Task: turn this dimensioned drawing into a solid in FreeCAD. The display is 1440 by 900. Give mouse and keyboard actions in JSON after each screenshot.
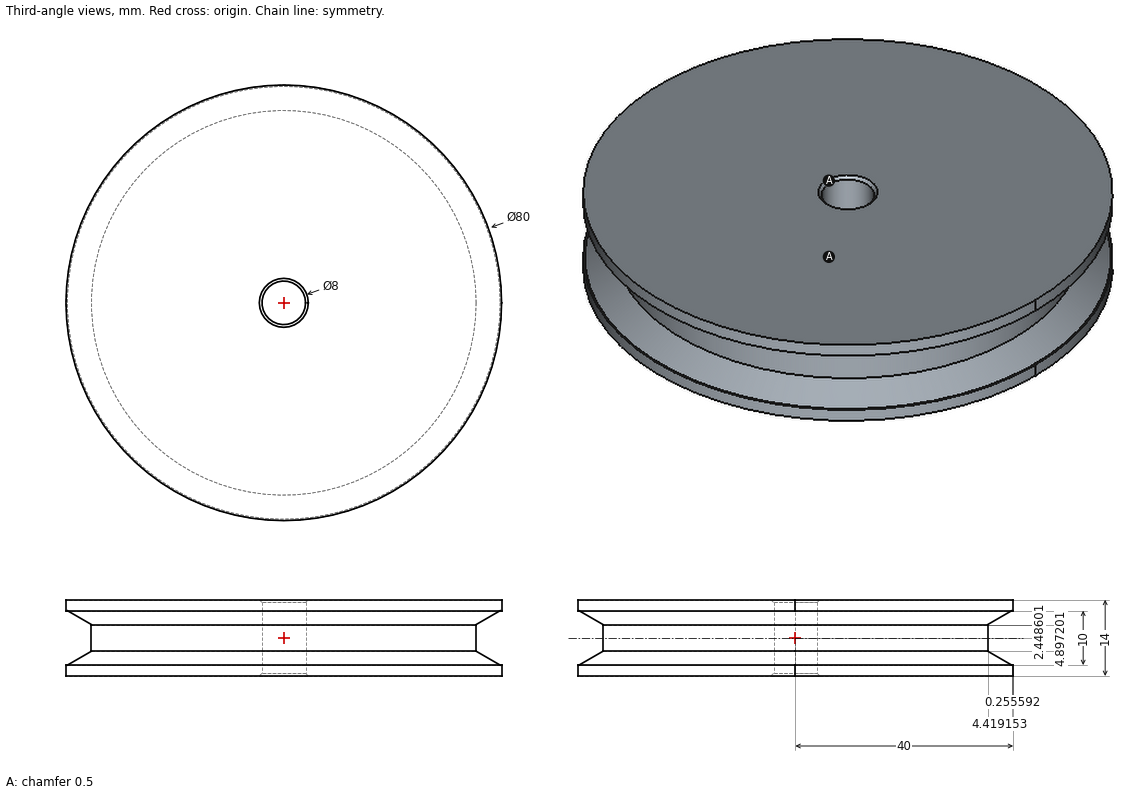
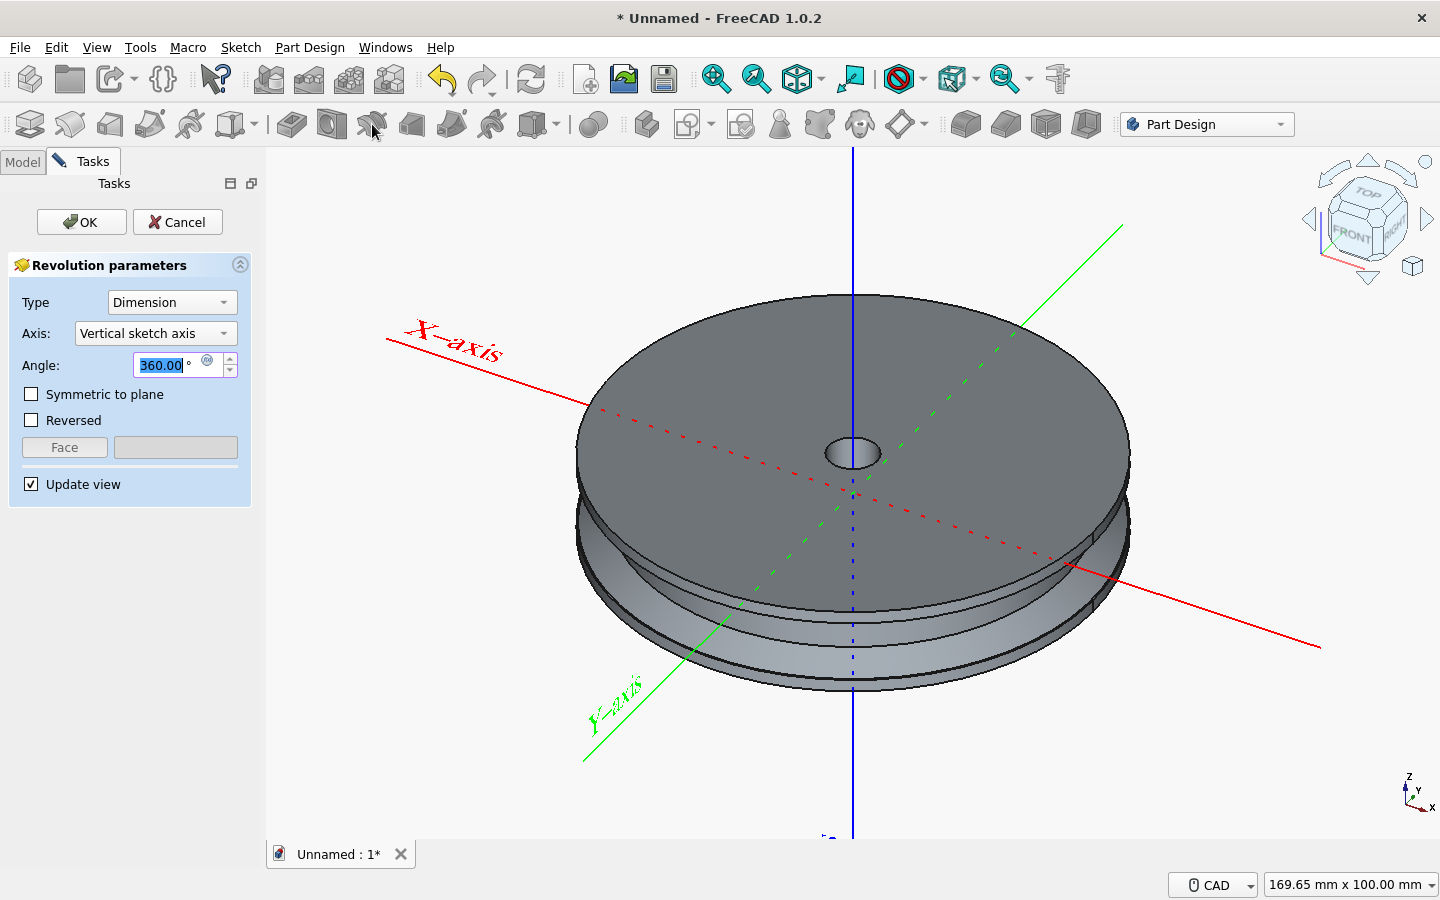
{"action": "left_click", "coordinate": [82, 222]}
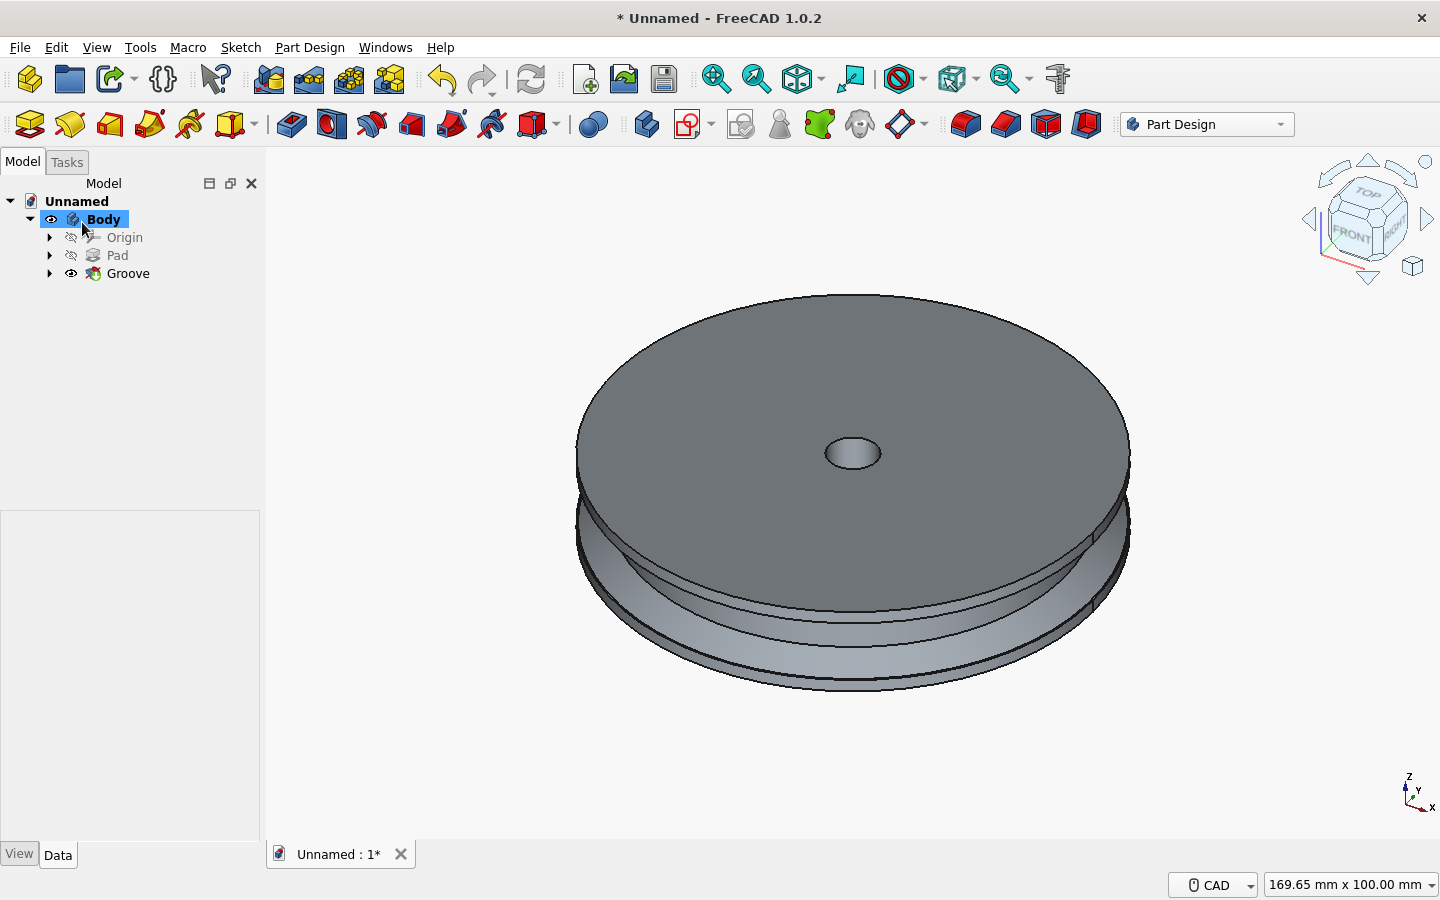
{"action": "left_click", "coordinate": [829, 444]}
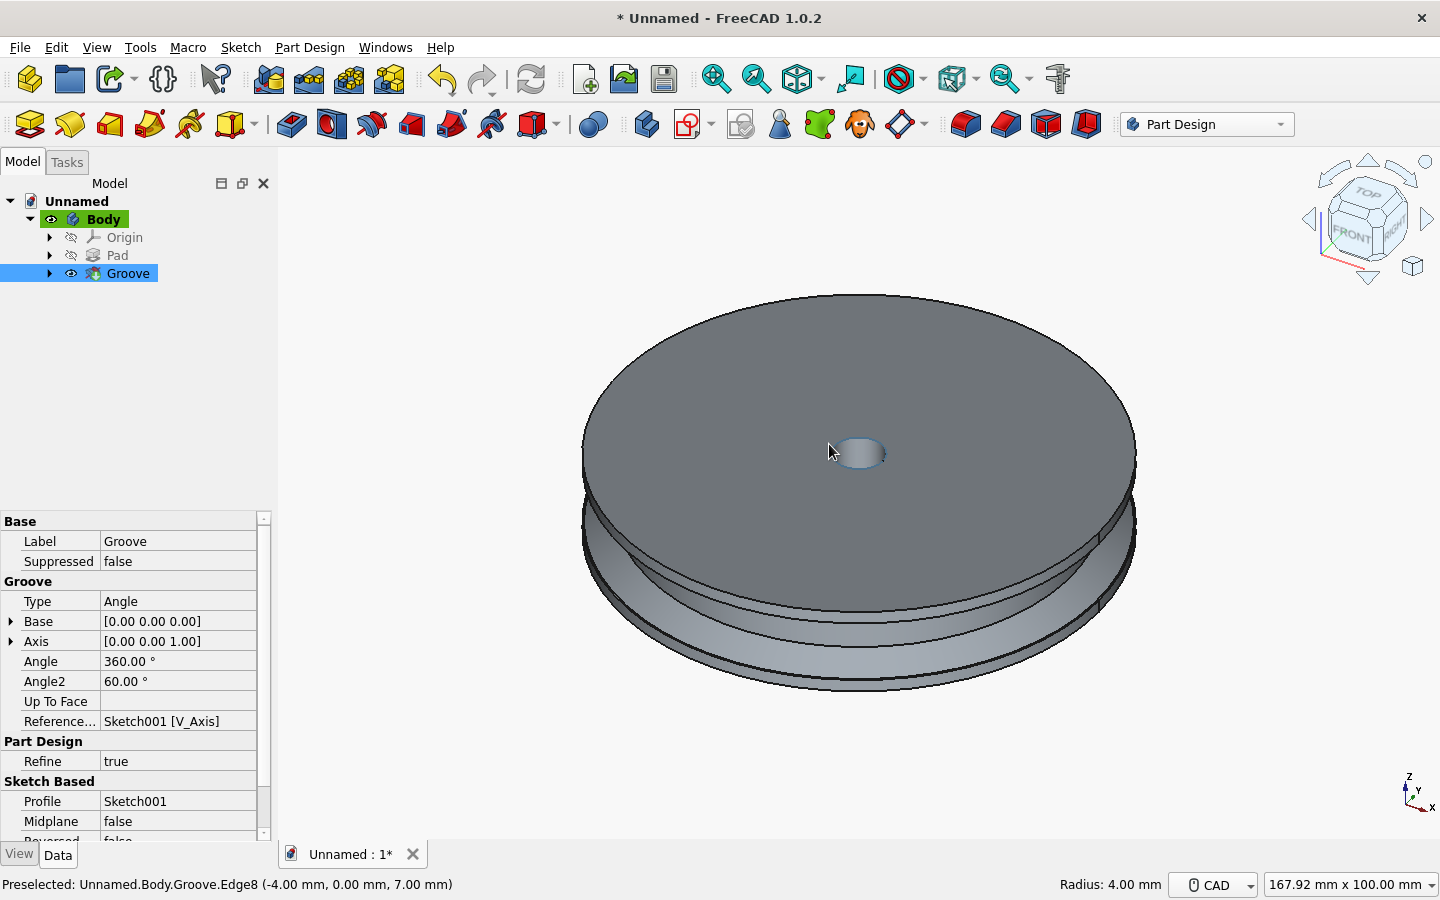
{"action": "key", "text": "0"}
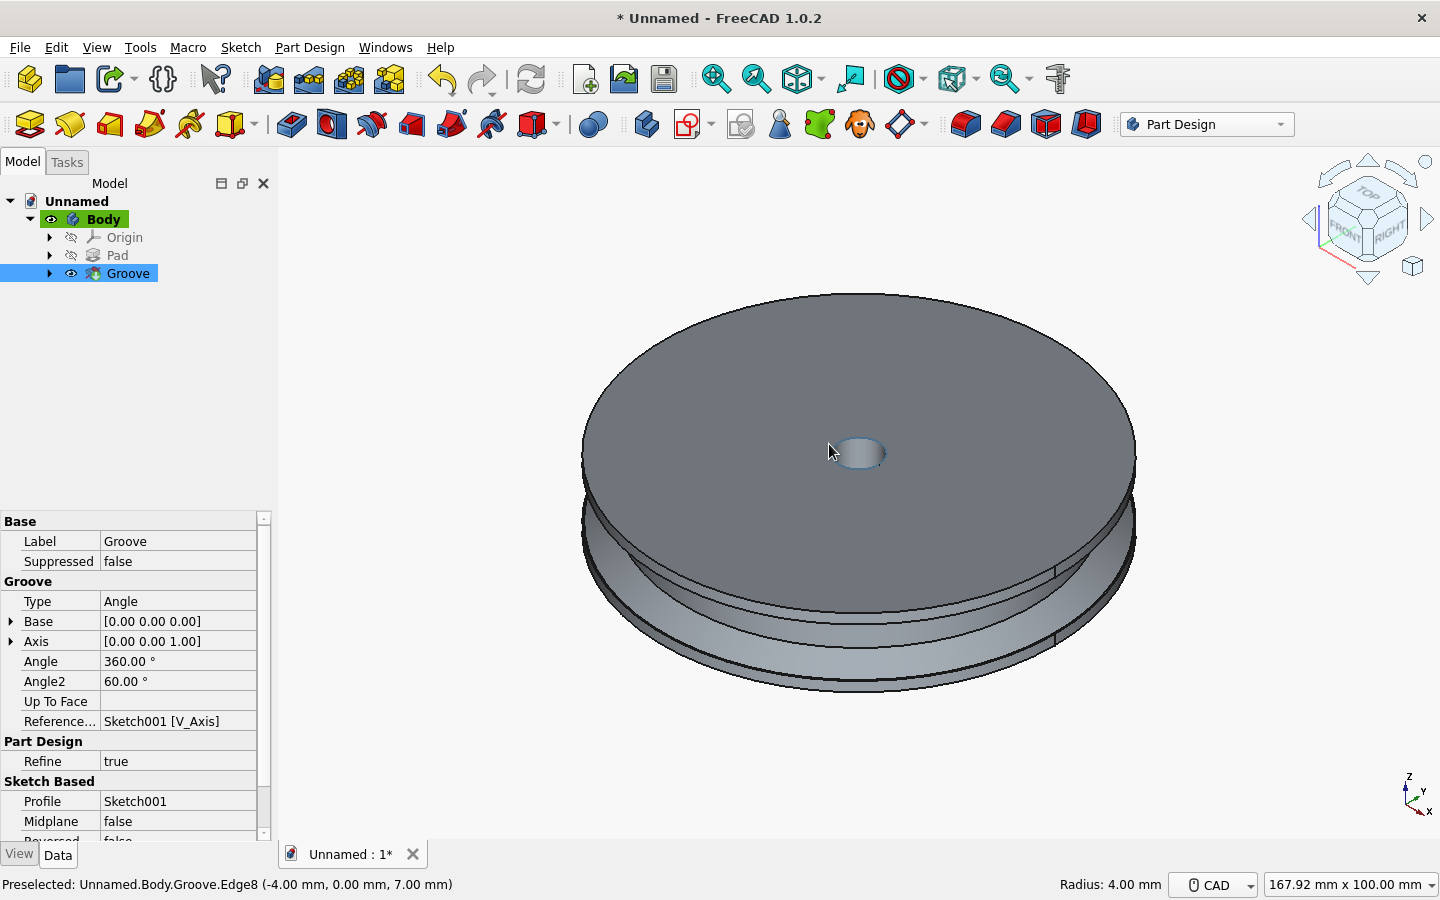
{"action": "key", "text": "2"}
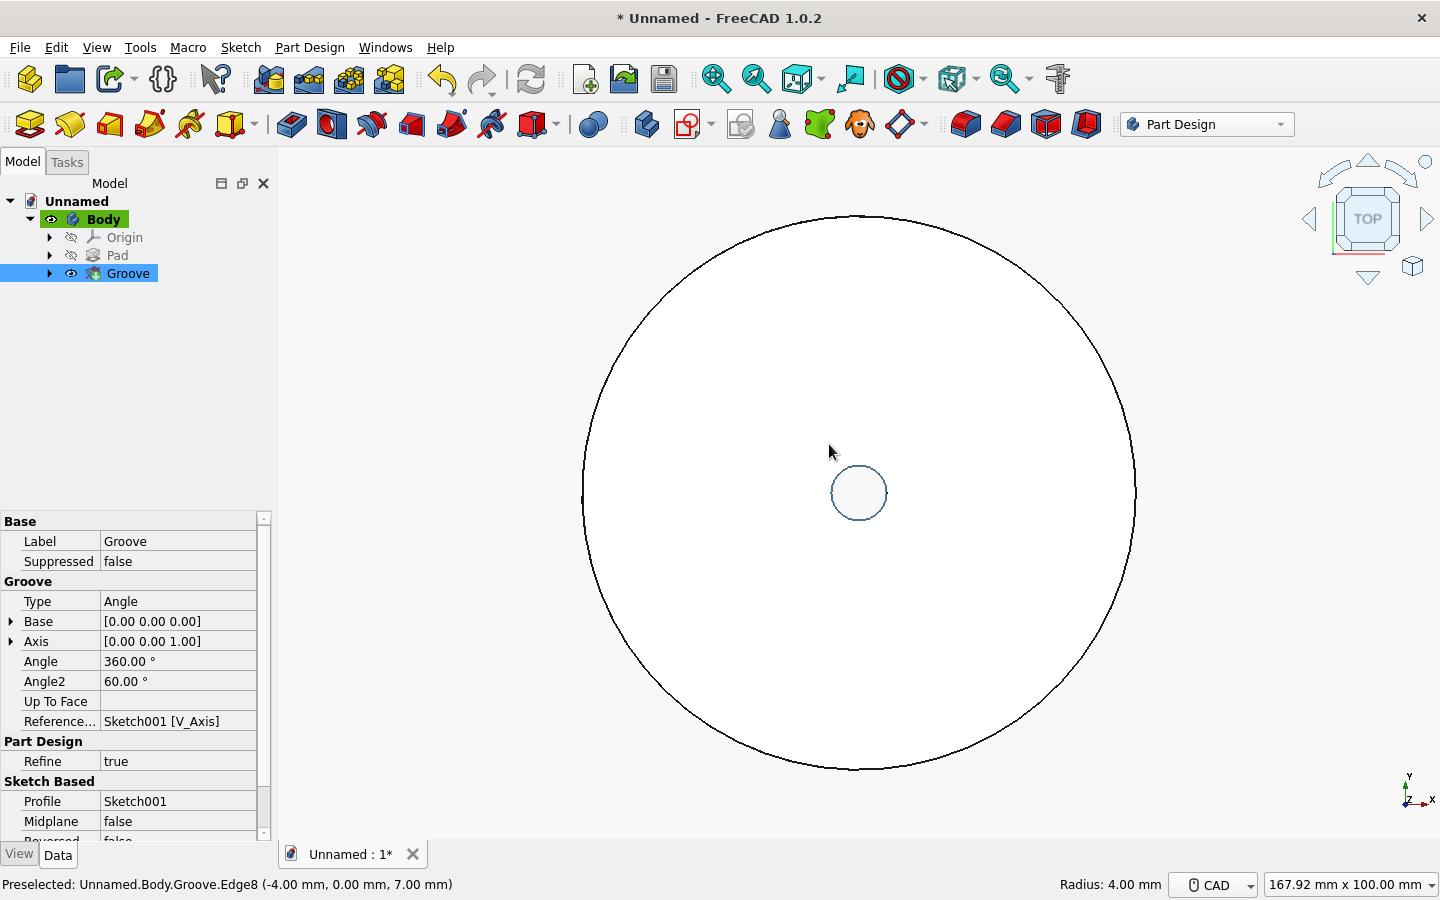
{"action": "key", "text": "1"}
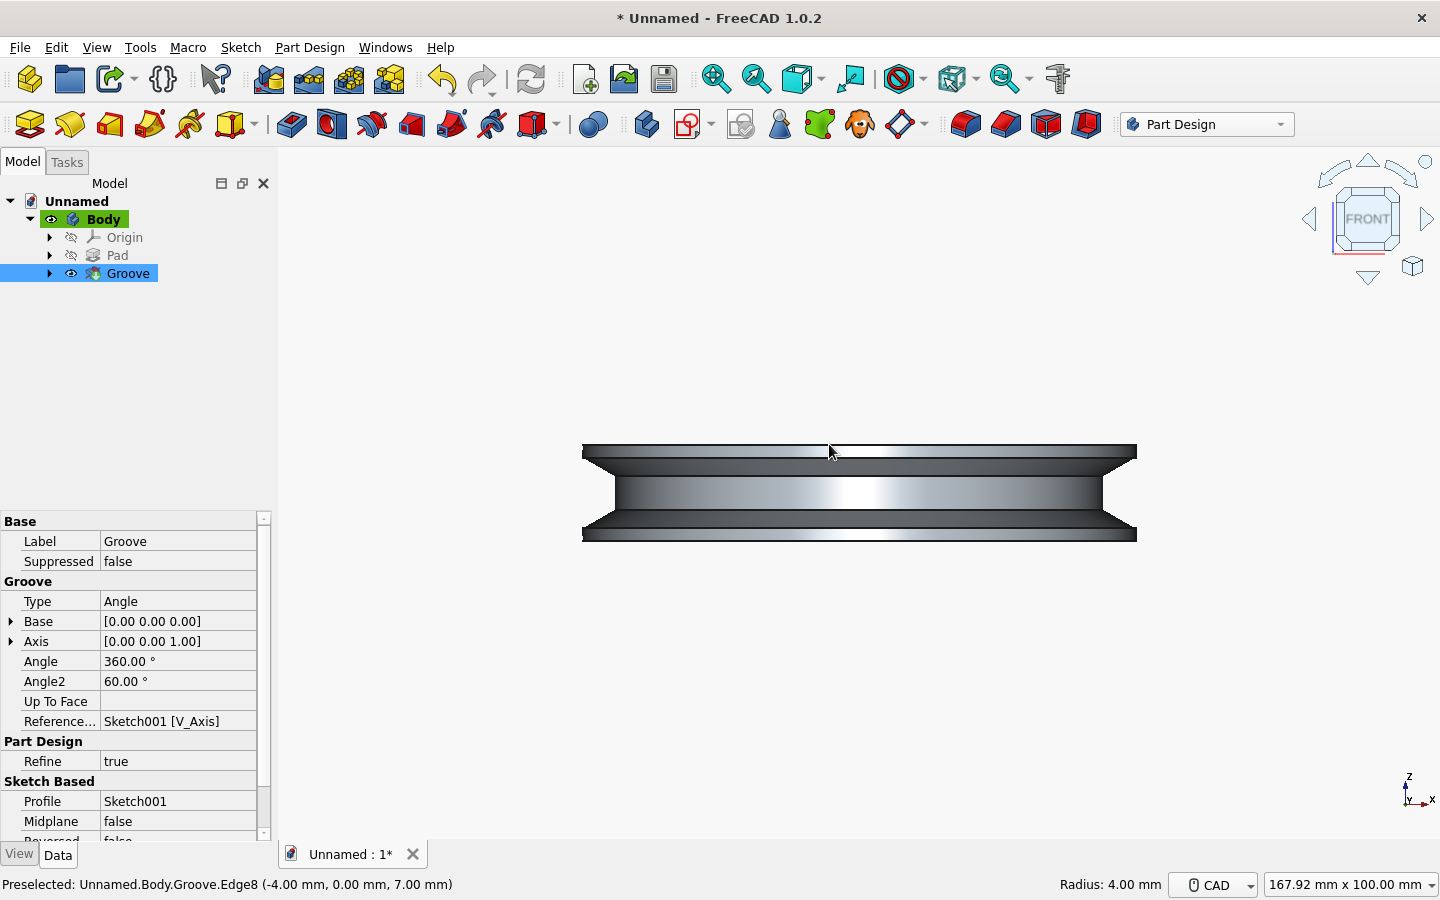
{"action": "key", "text": "3"}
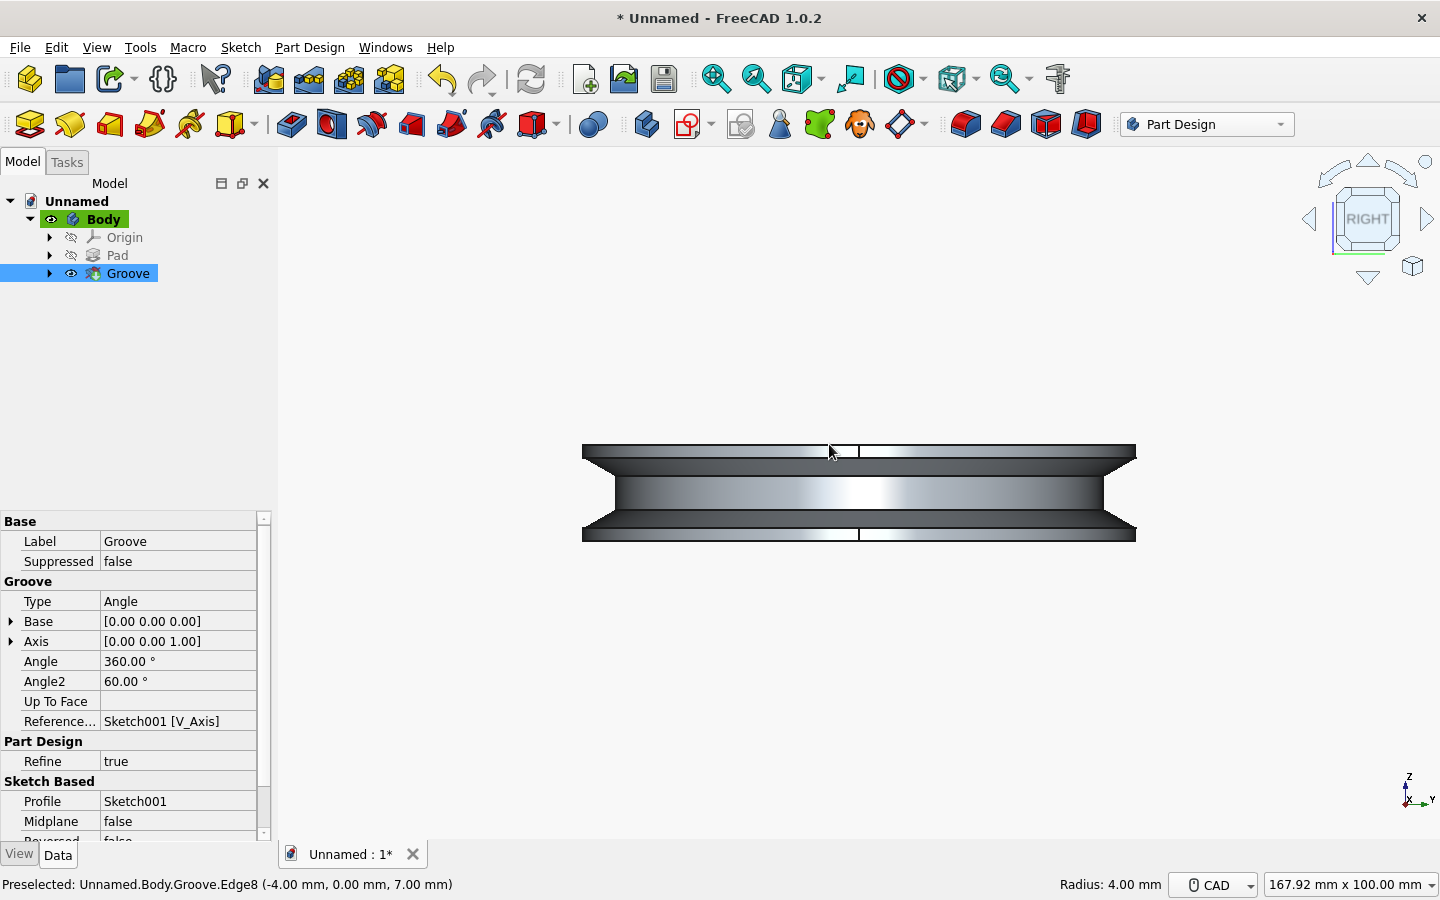
{"action": "key", "text": "5"}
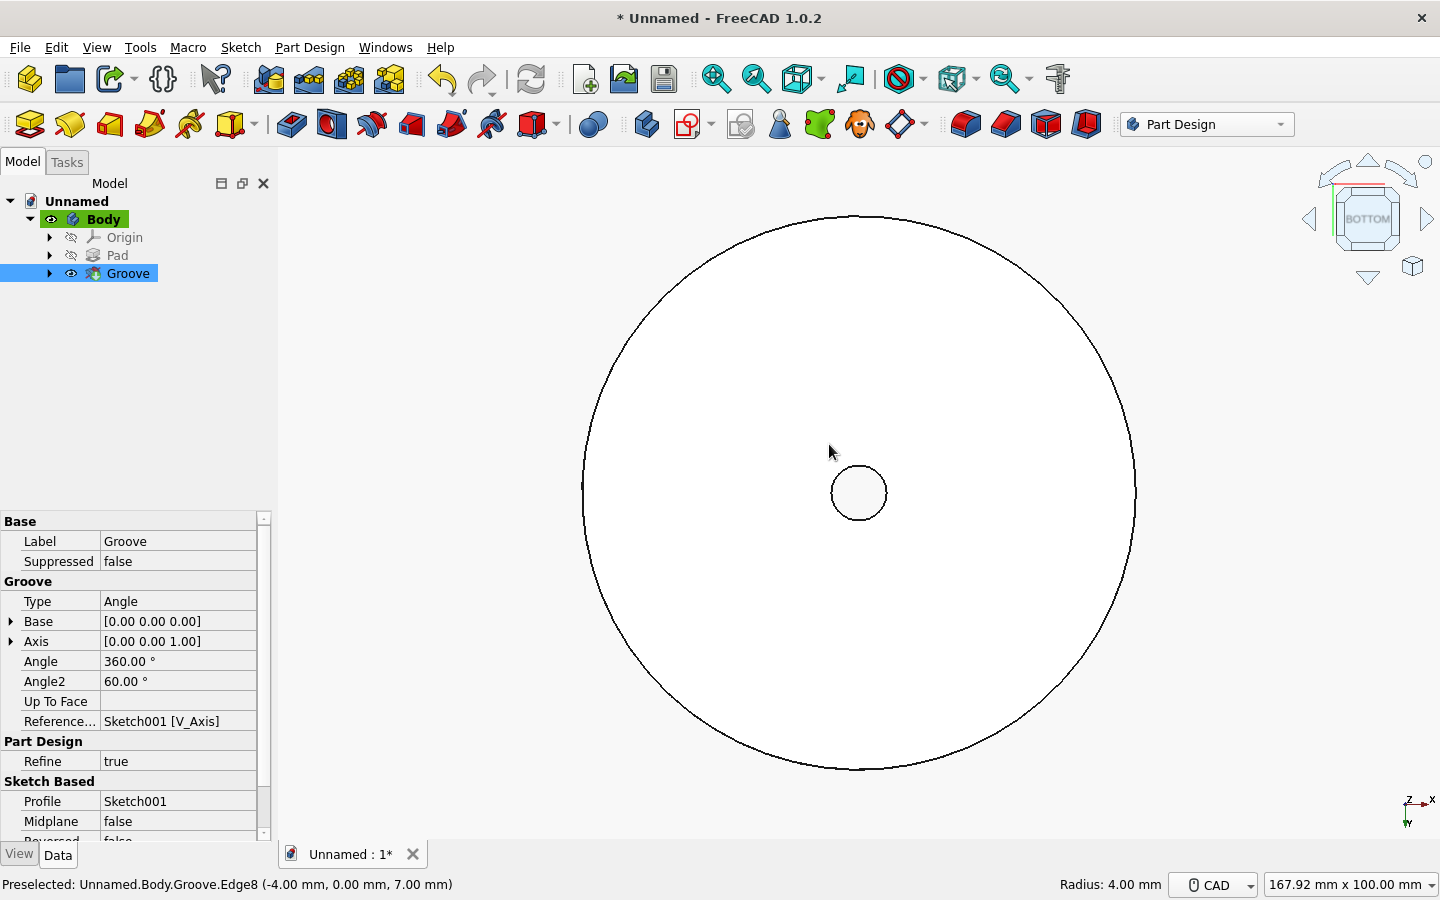
{"action": "left_click", "coordinate": [831, 492], "text": "ctrl"}